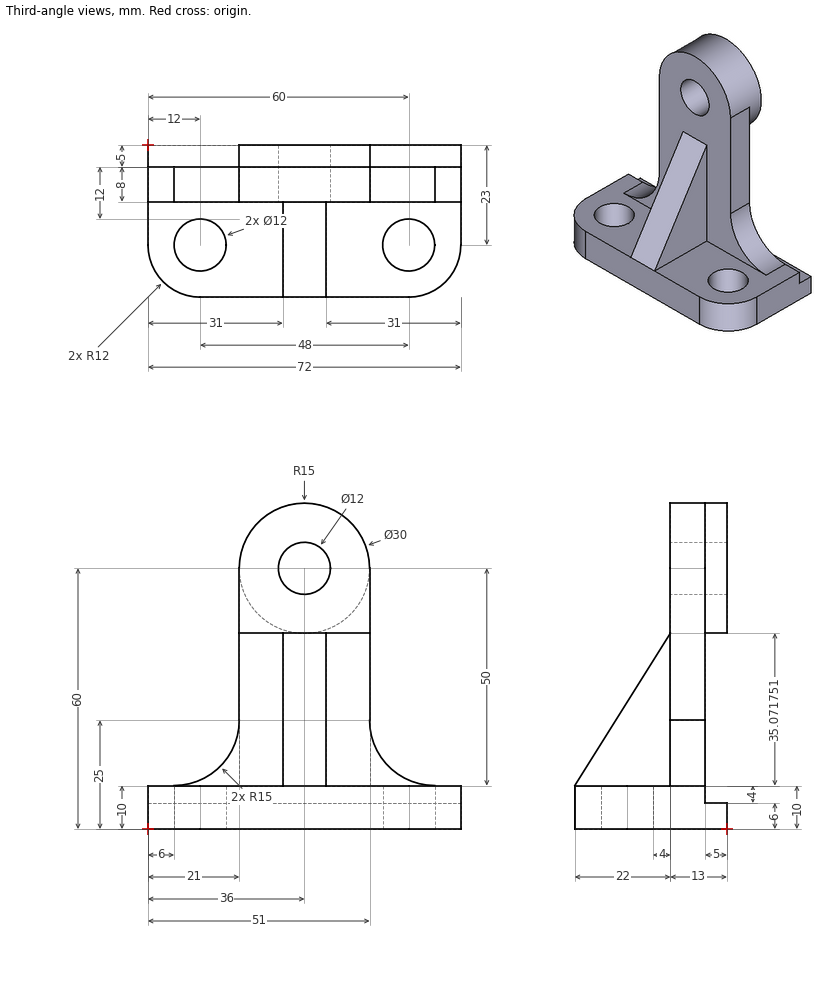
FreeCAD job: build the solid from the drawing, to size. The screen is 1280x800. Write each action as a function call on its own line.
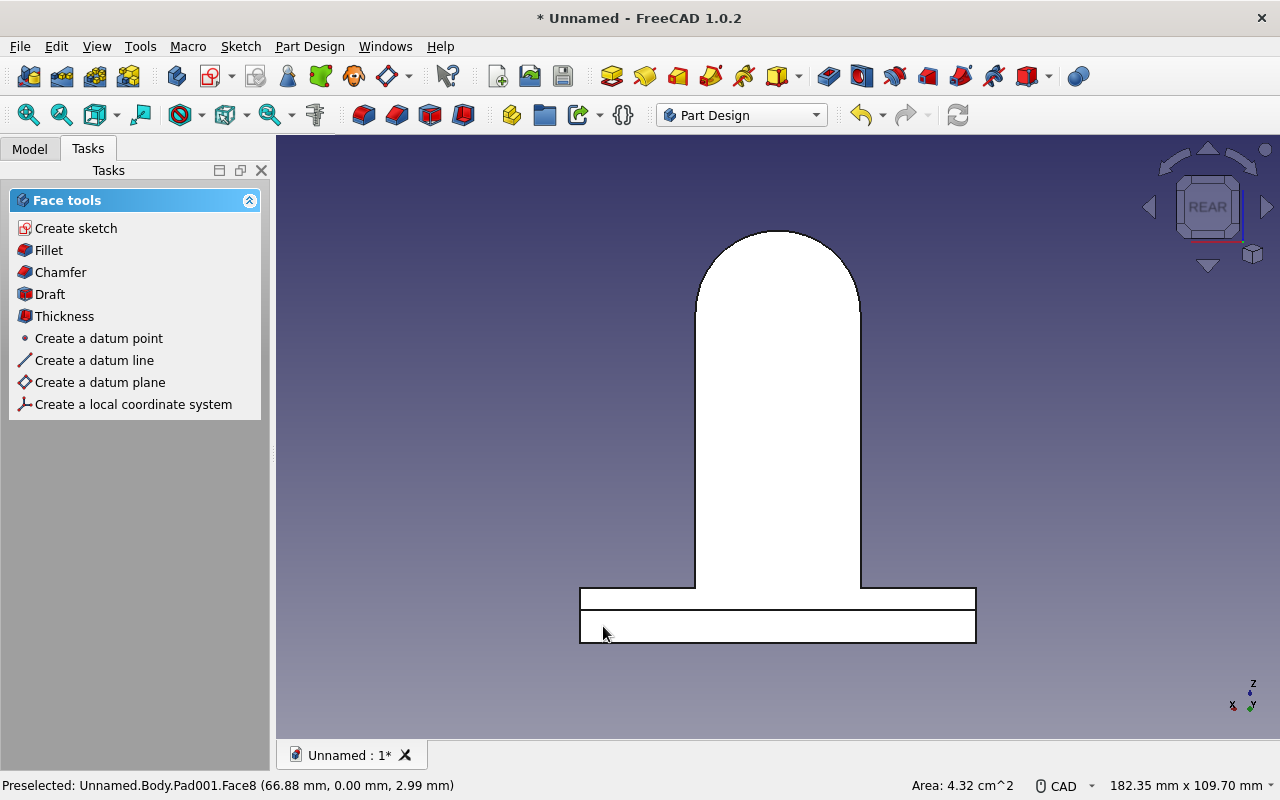
click(210, 76)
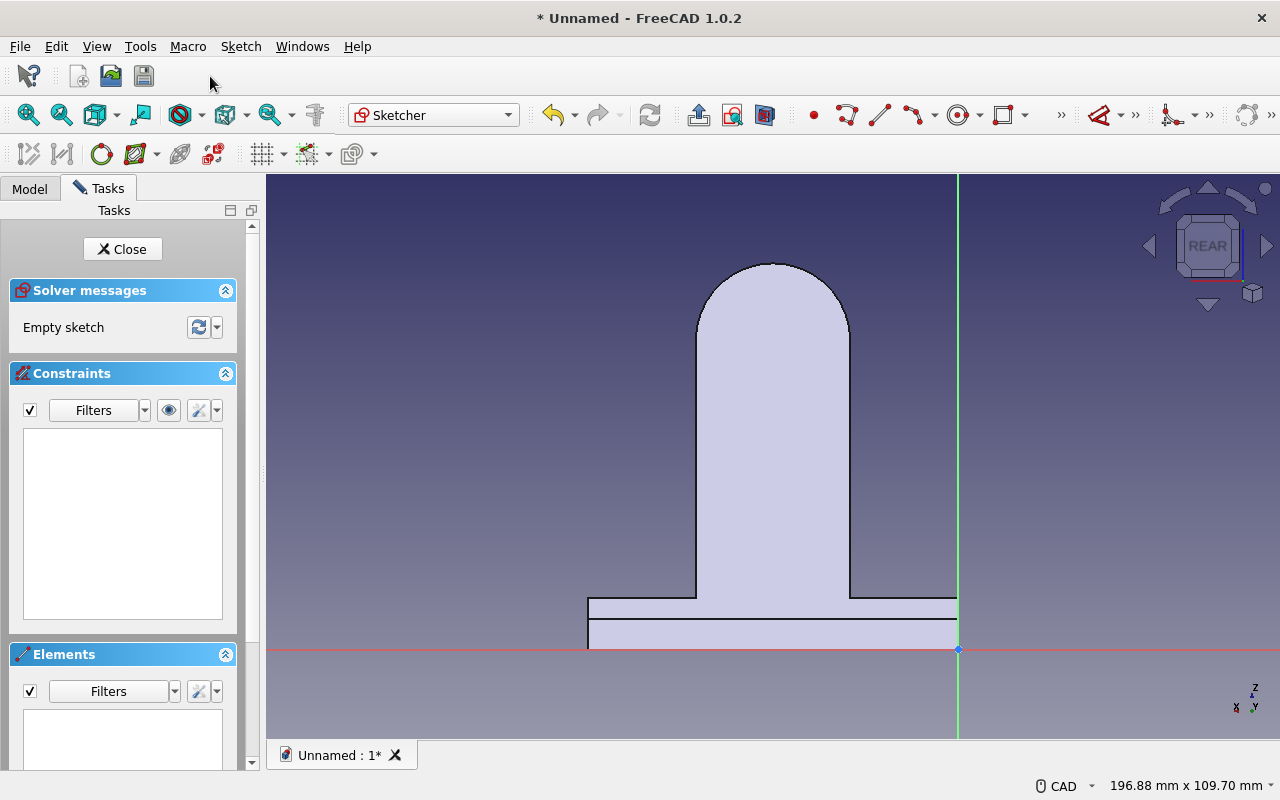
scroll(829, 246, up, 4)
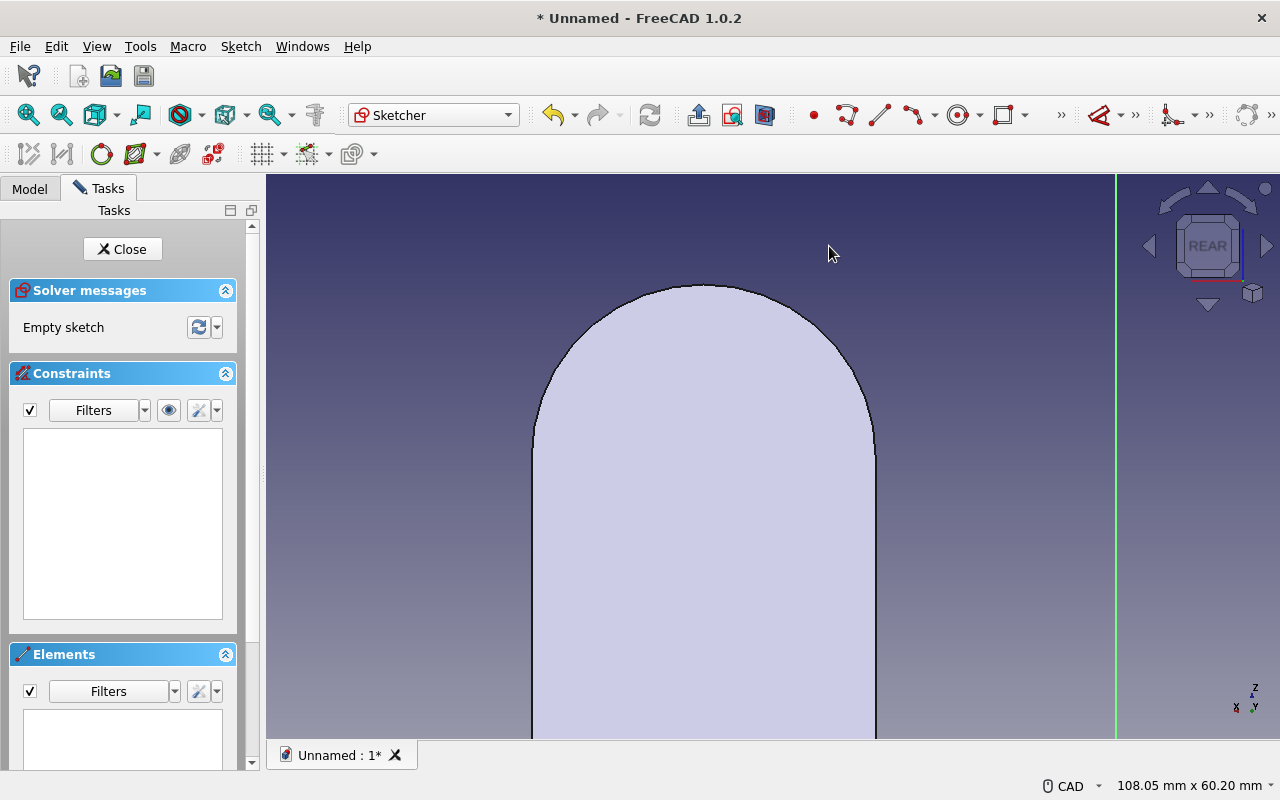
key(g)
key(c)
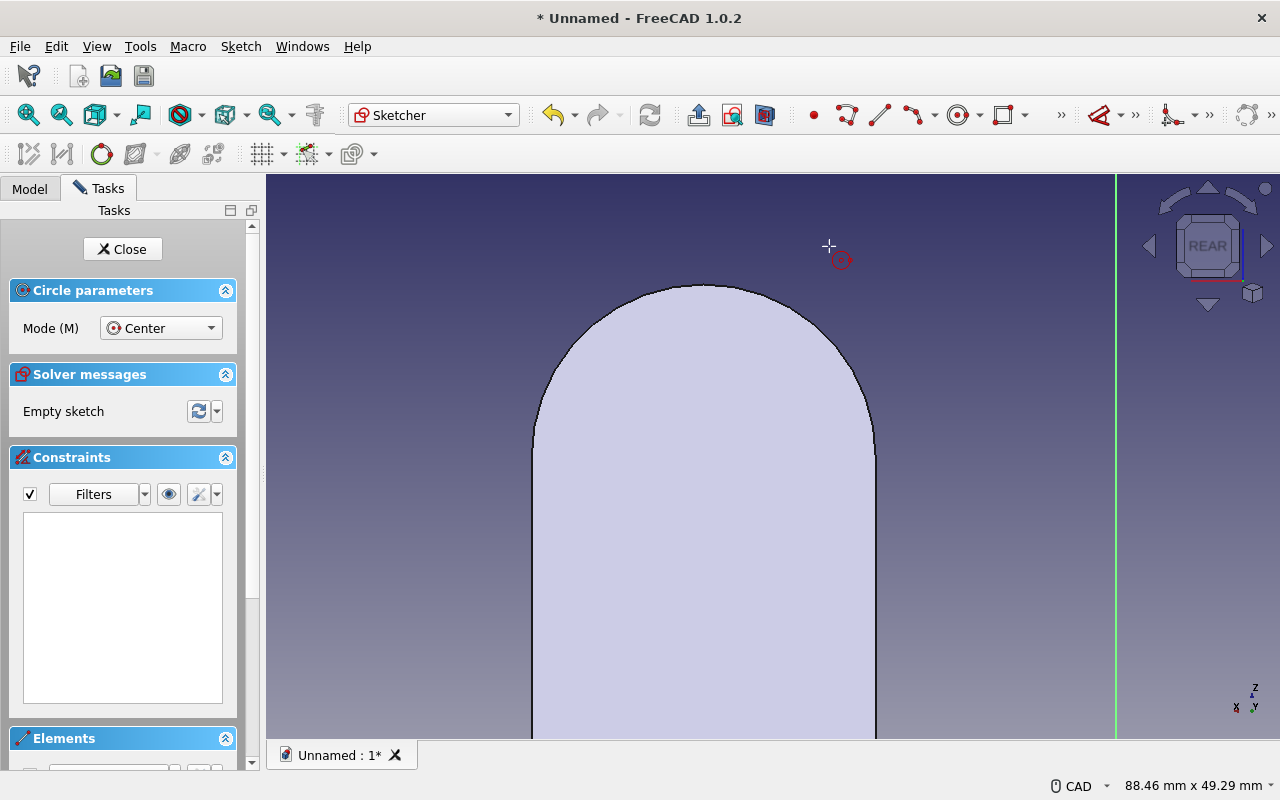
click(704, 456)
click(825, 335)
key(Escape)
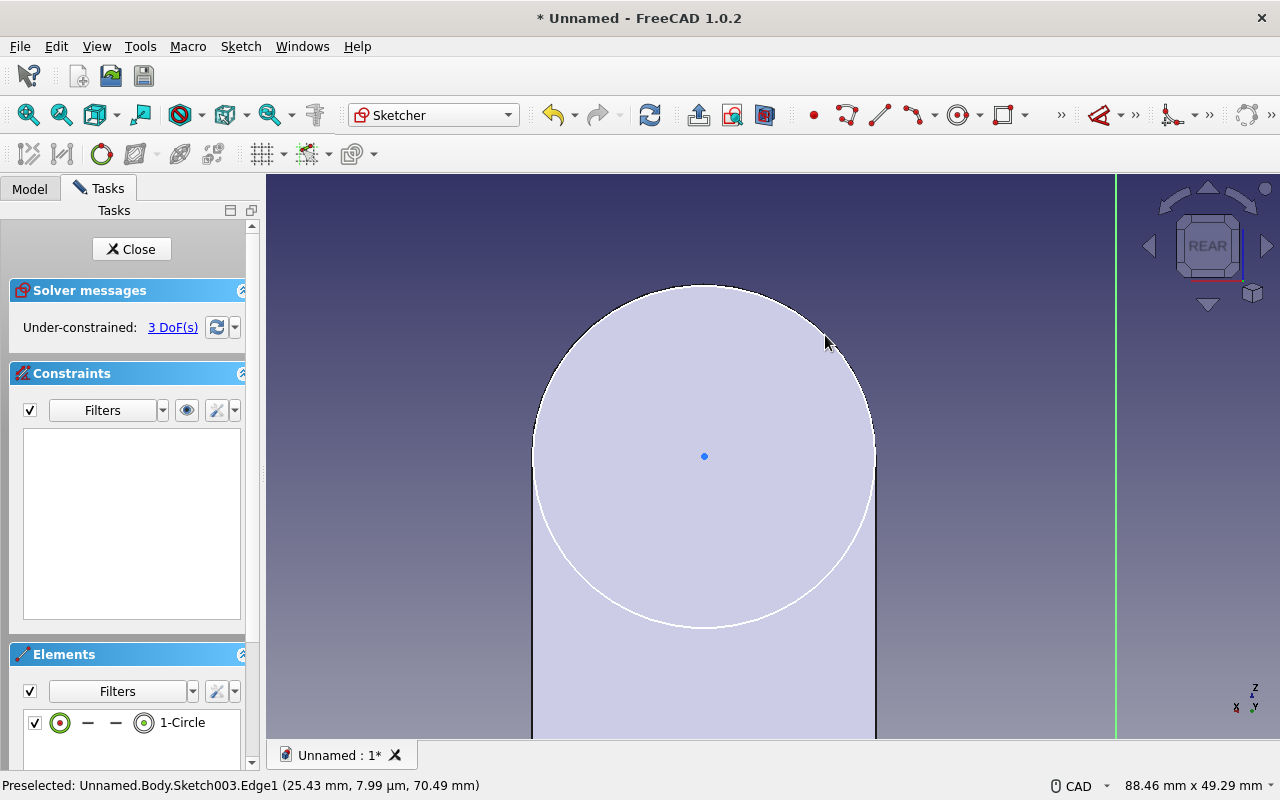
click(1098, 116)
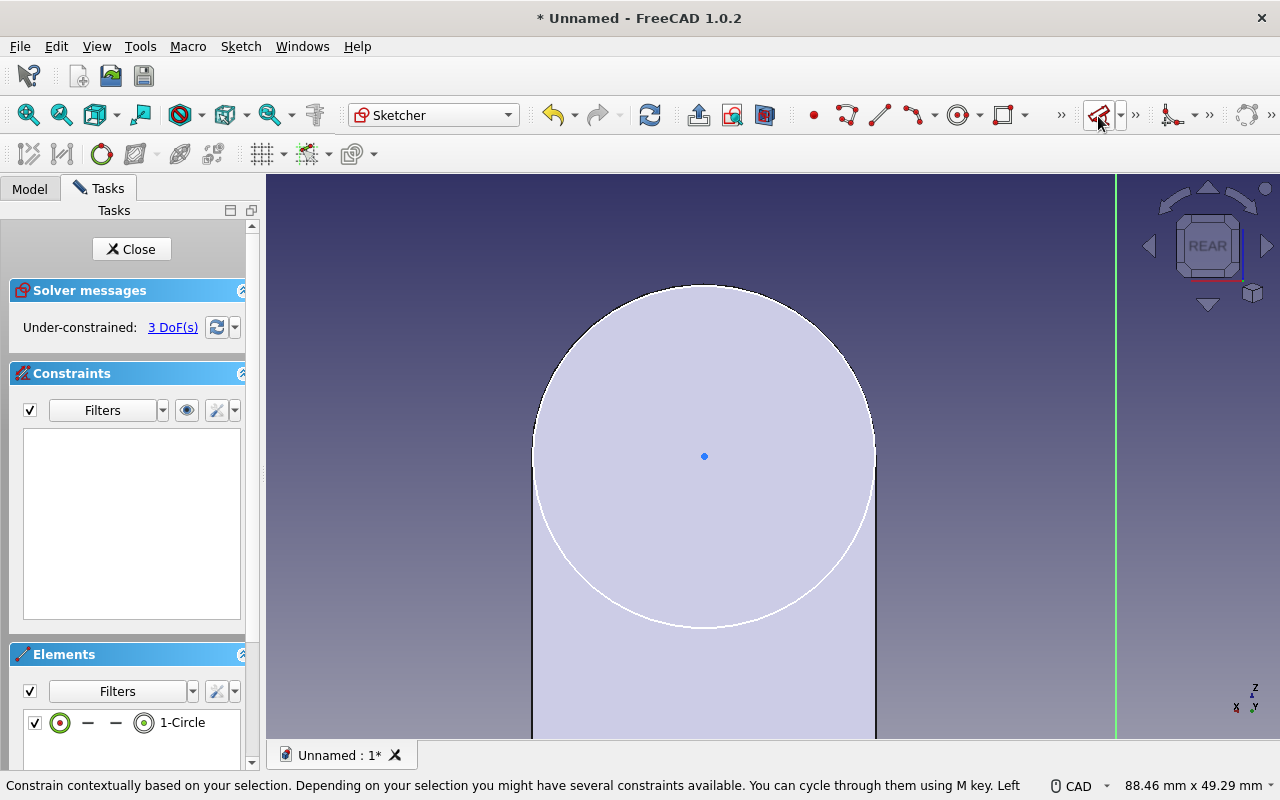
click(825, 336)
click(848, 313)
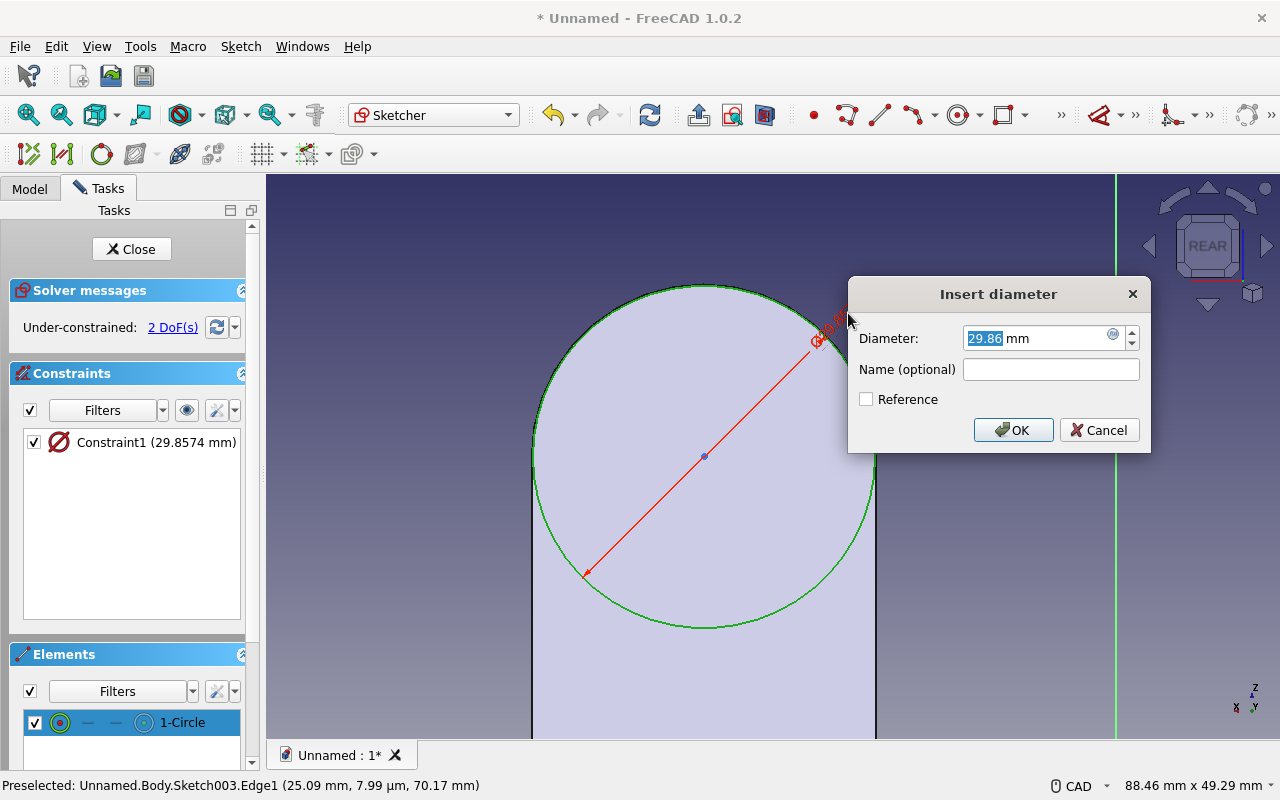
text(30)
key(Return)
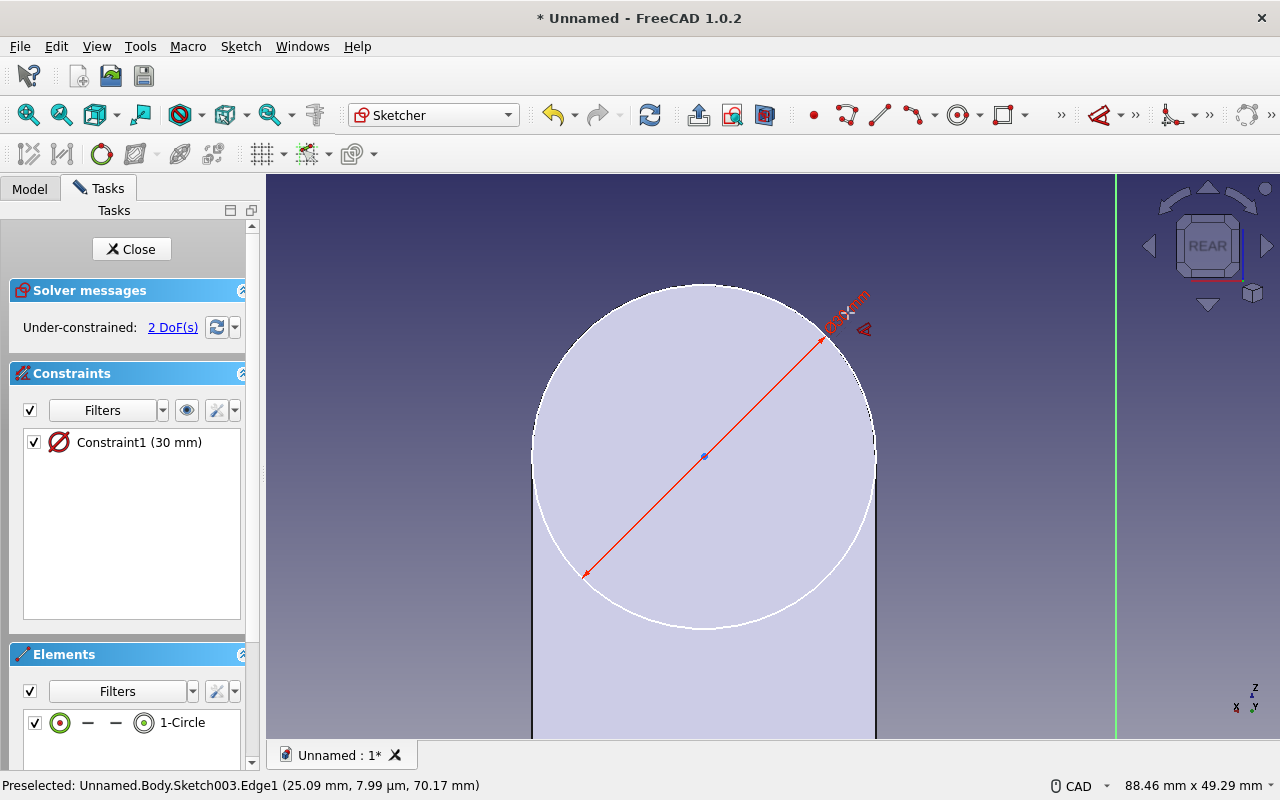
click(704, 457)
click(910, 423)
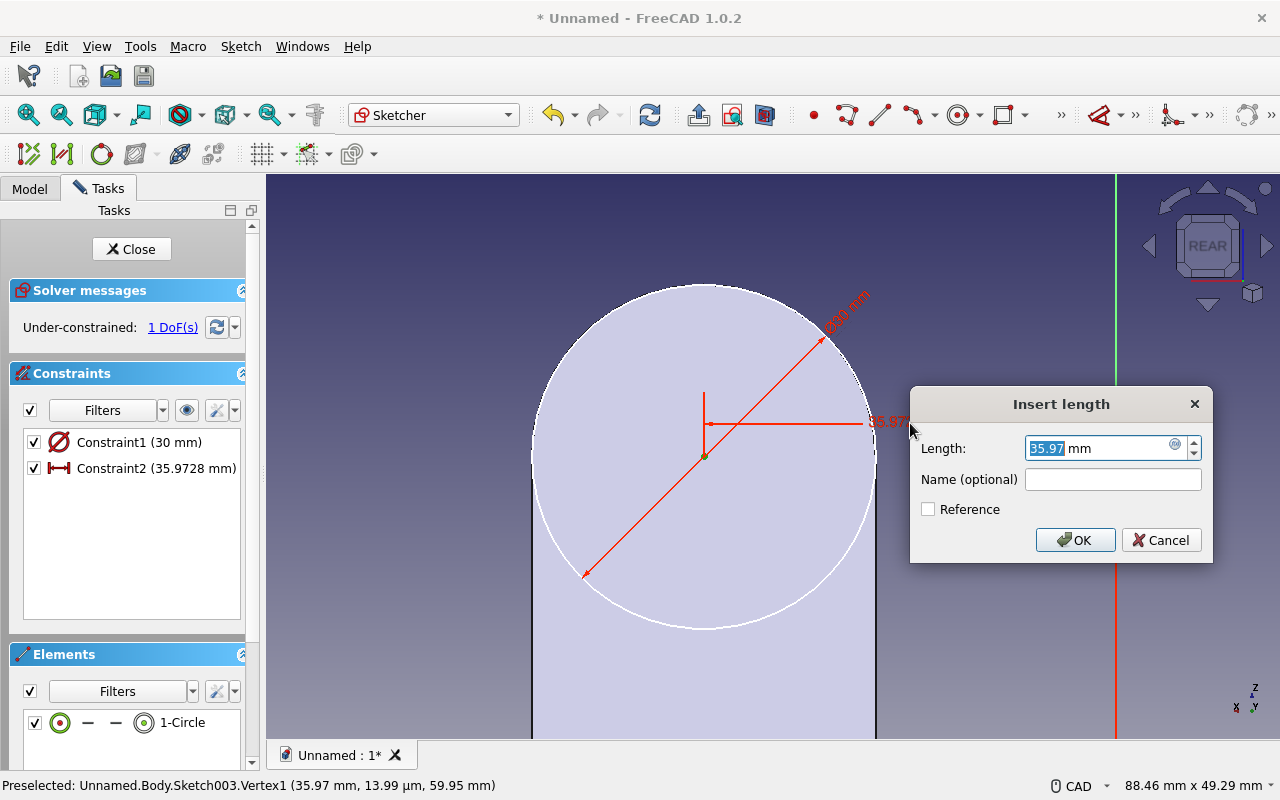
text(36)
key(Return)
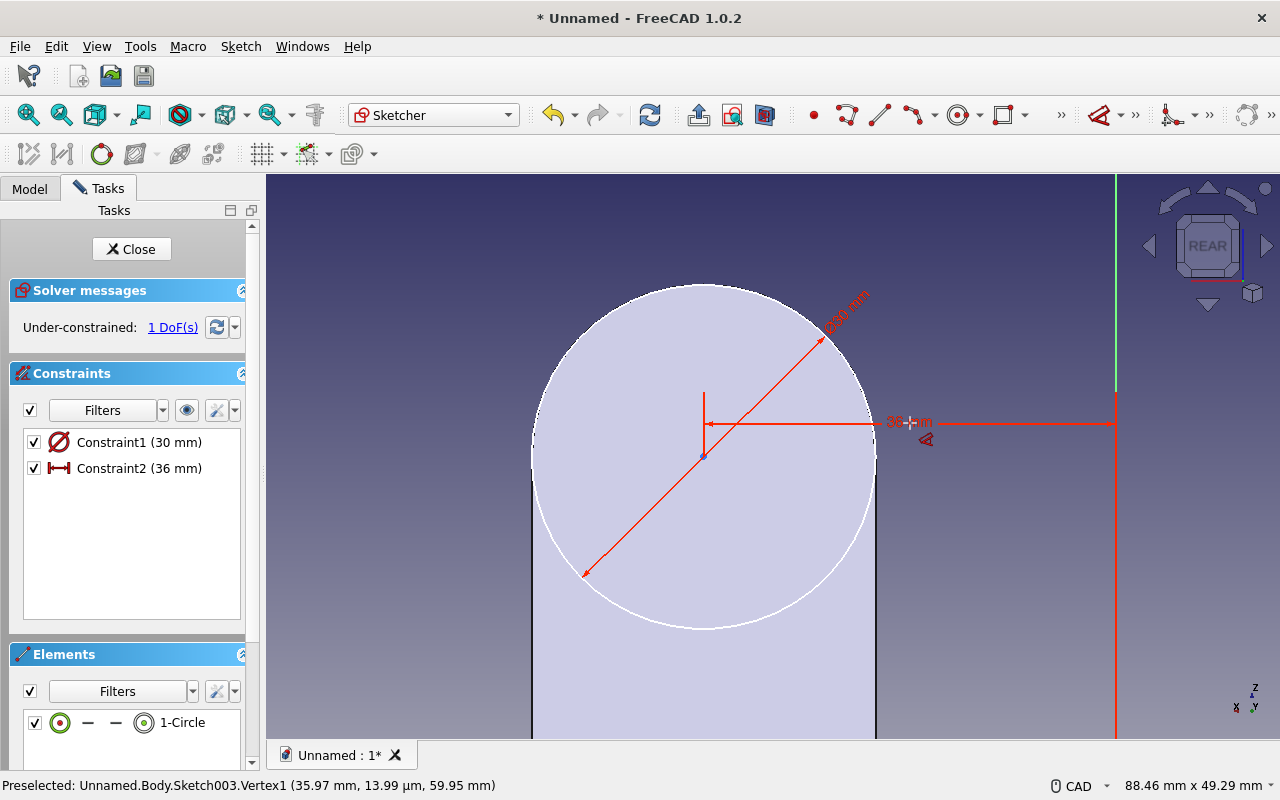
click(704, 457)
click(670, 584)